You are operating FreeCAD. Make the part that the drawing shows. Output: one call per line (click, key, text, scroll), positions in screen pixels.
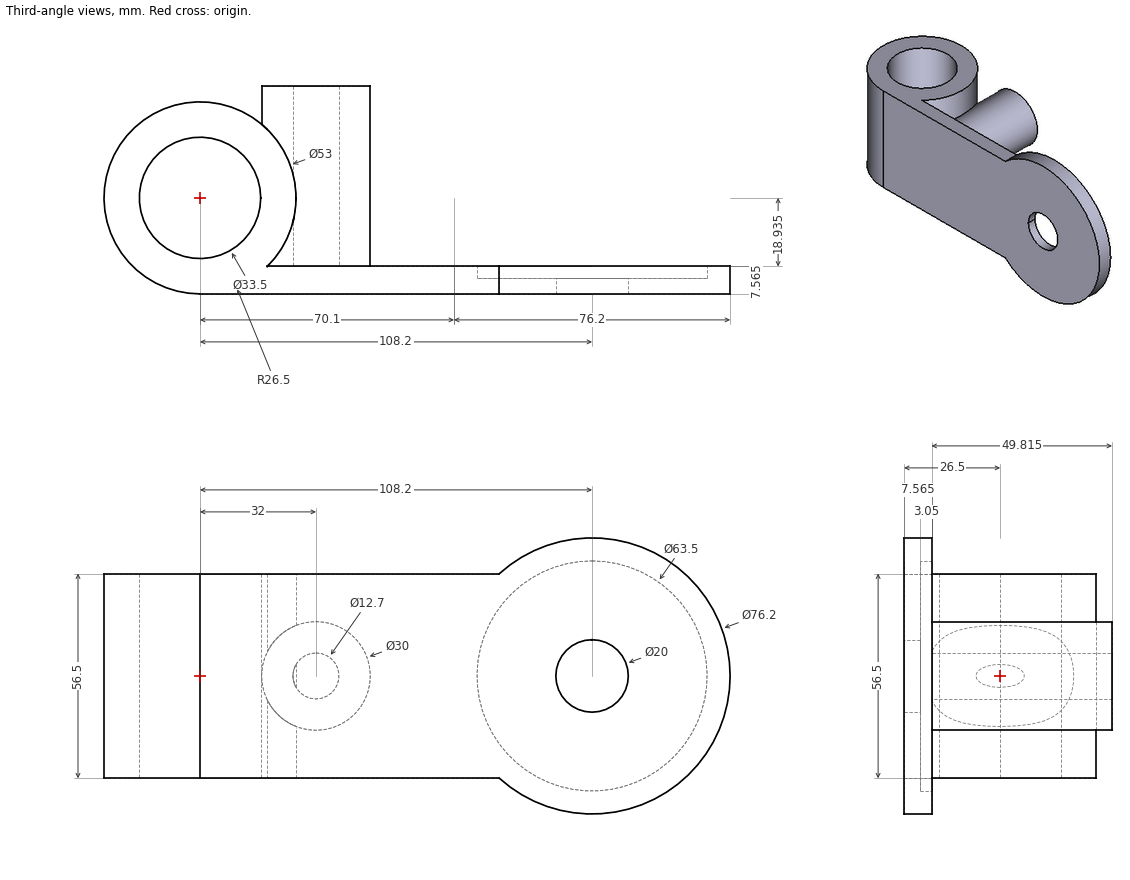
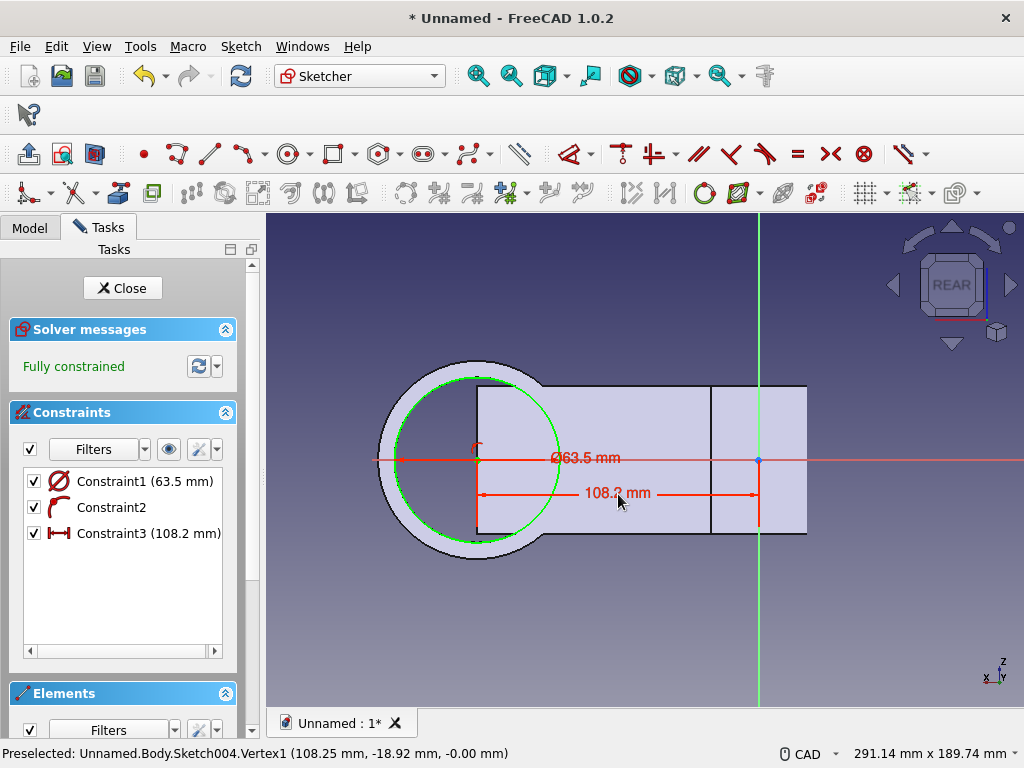
click(123, 288)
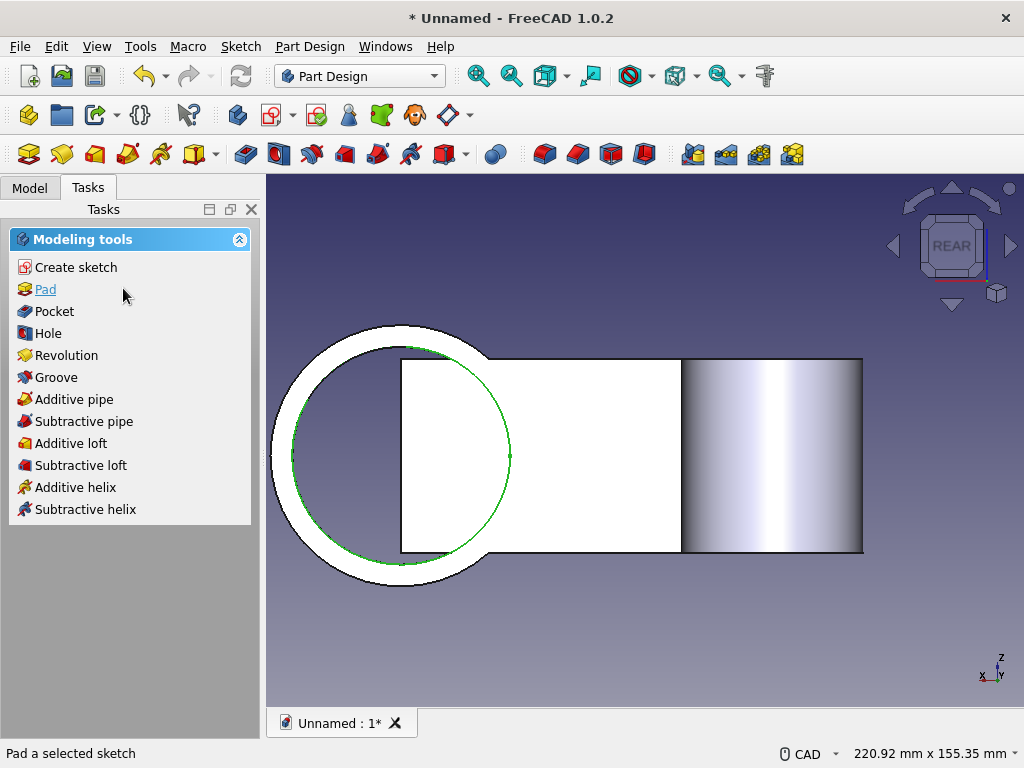
click(29, 154)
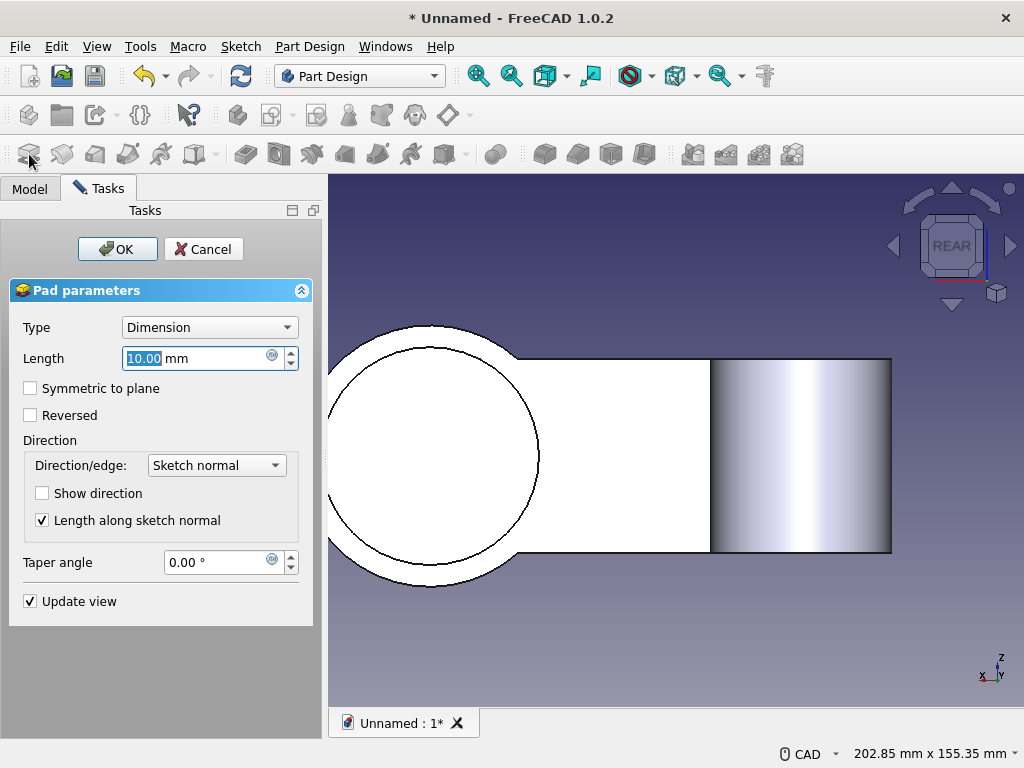
text(7.565)
key(Tab)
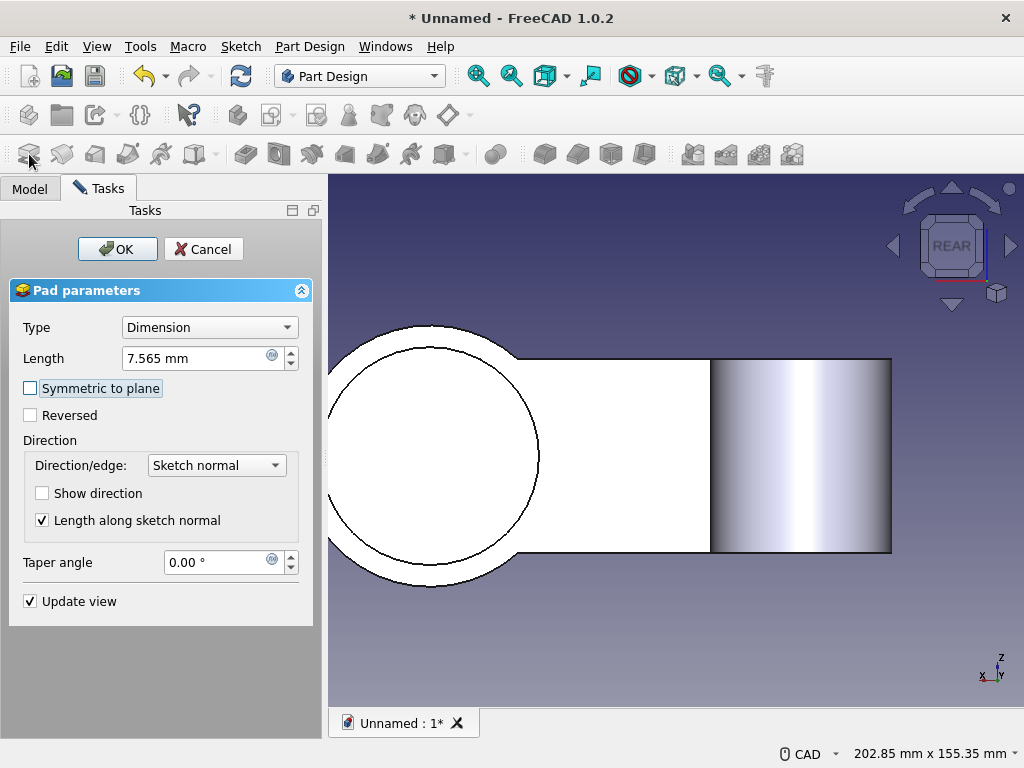
click(31, 415)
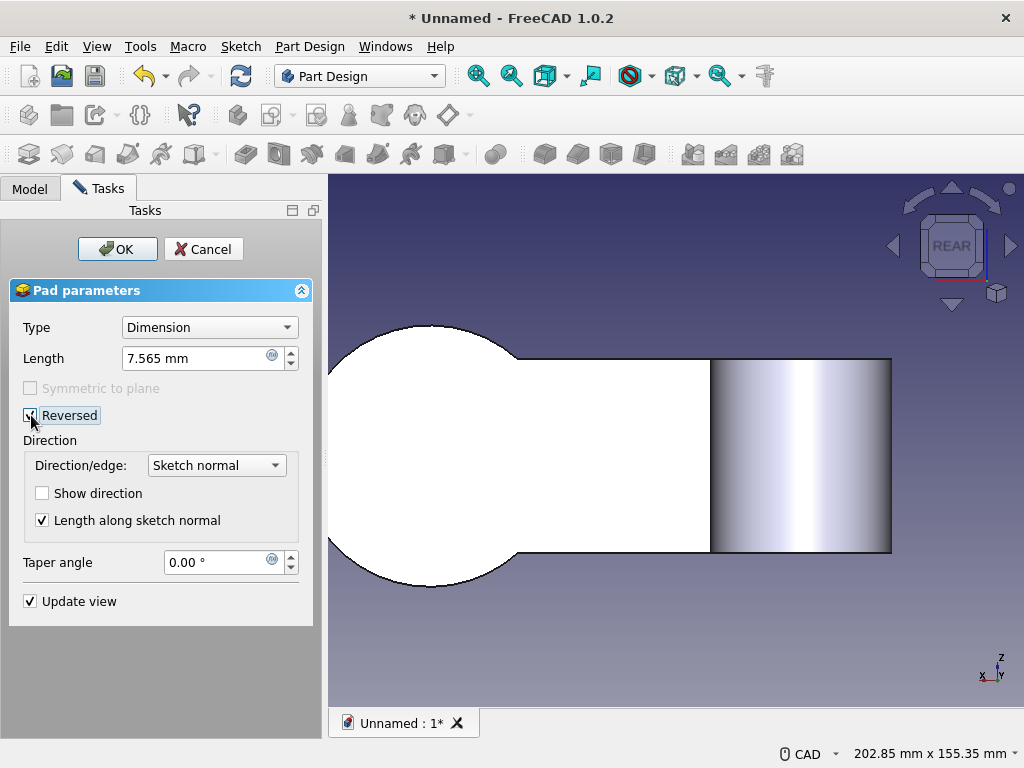
click(118, 249)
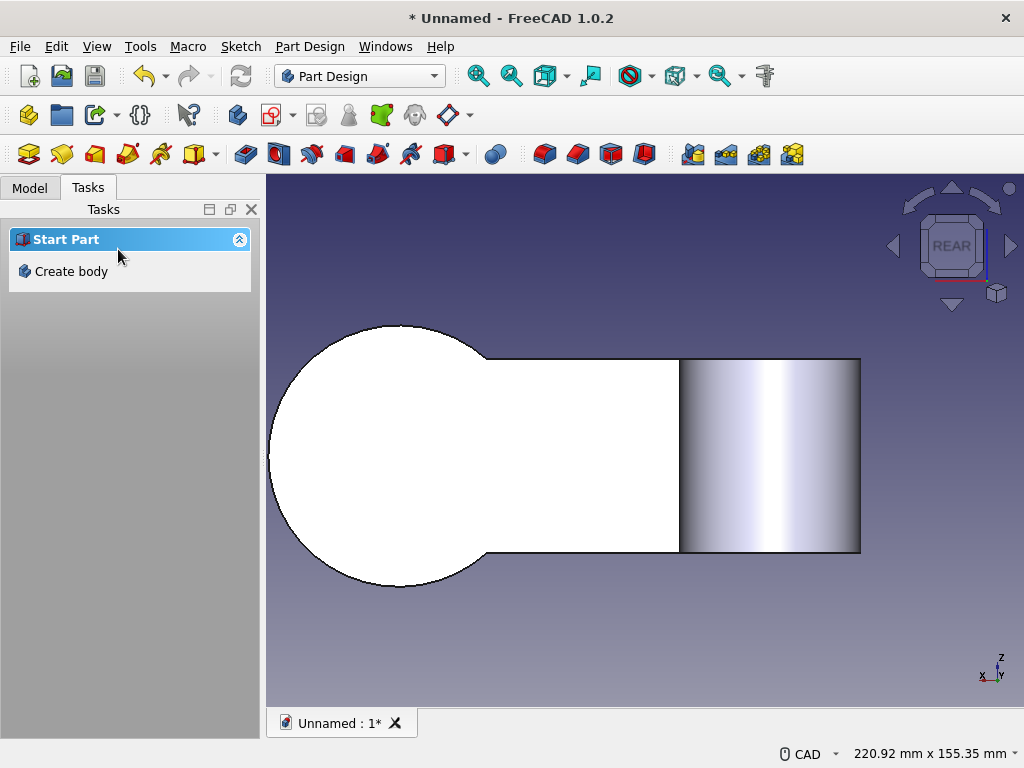
click(425, 455)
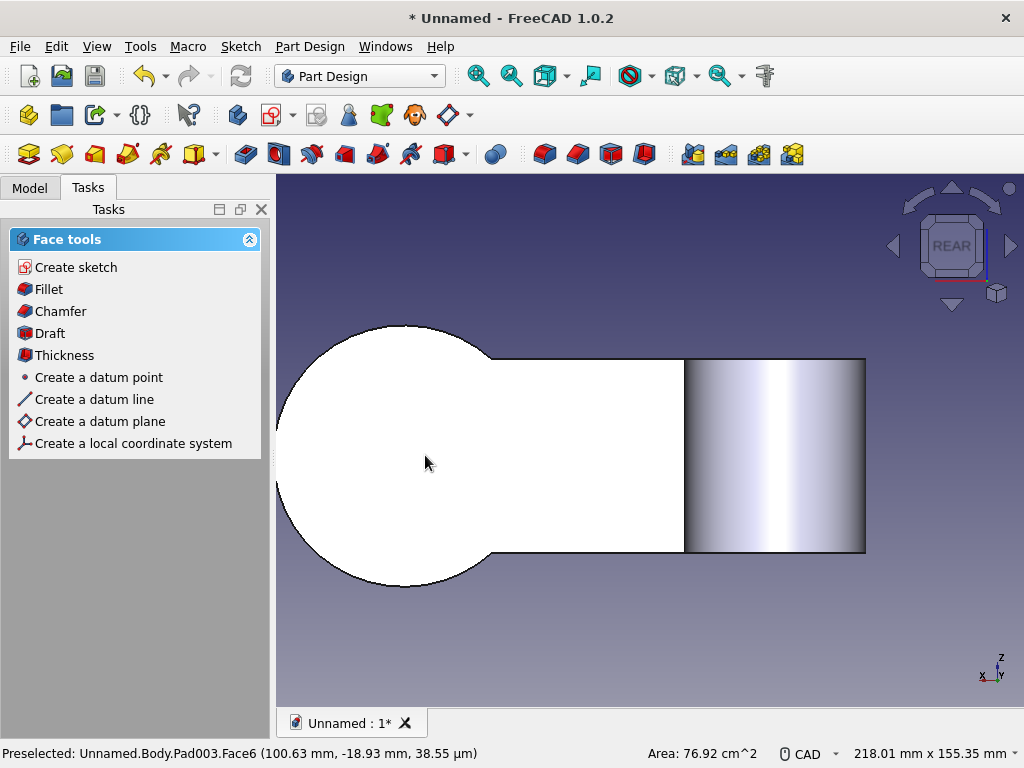
click(270, 116)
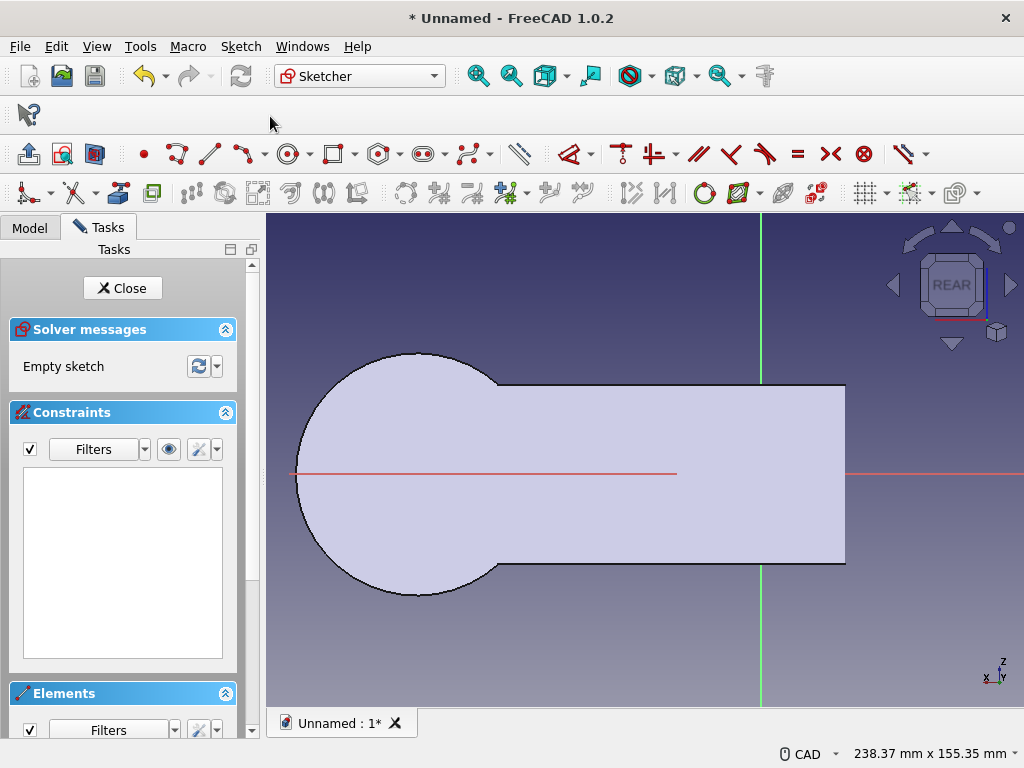
scroll(748, 395, down, 1)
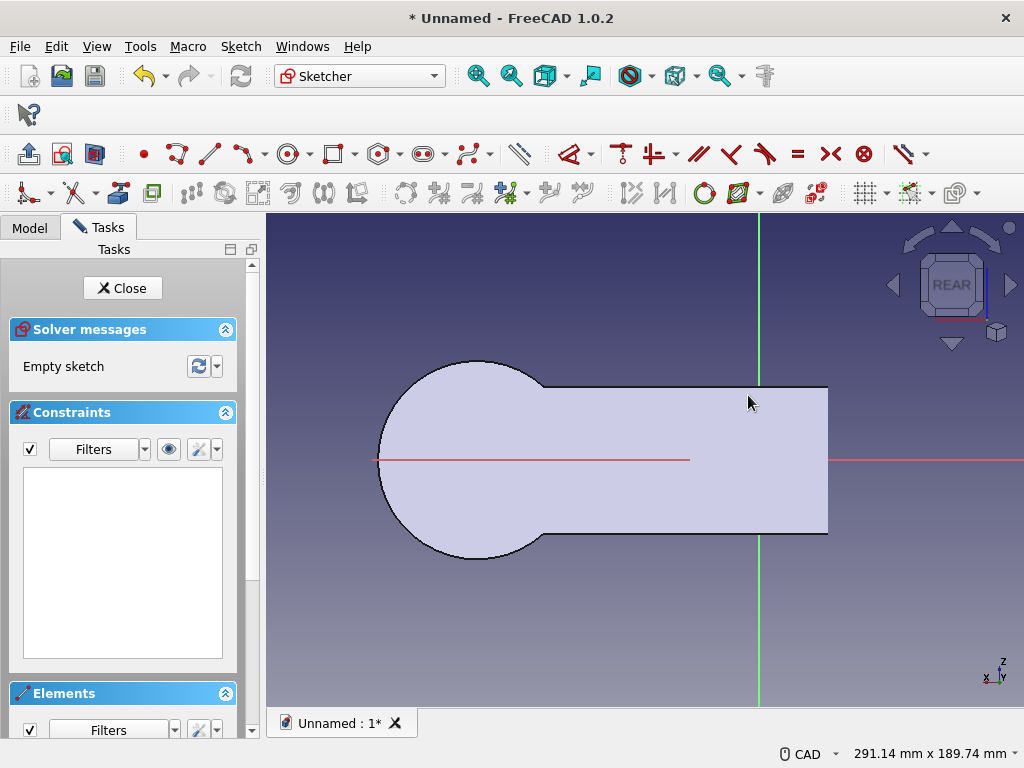
key(g)
key(c)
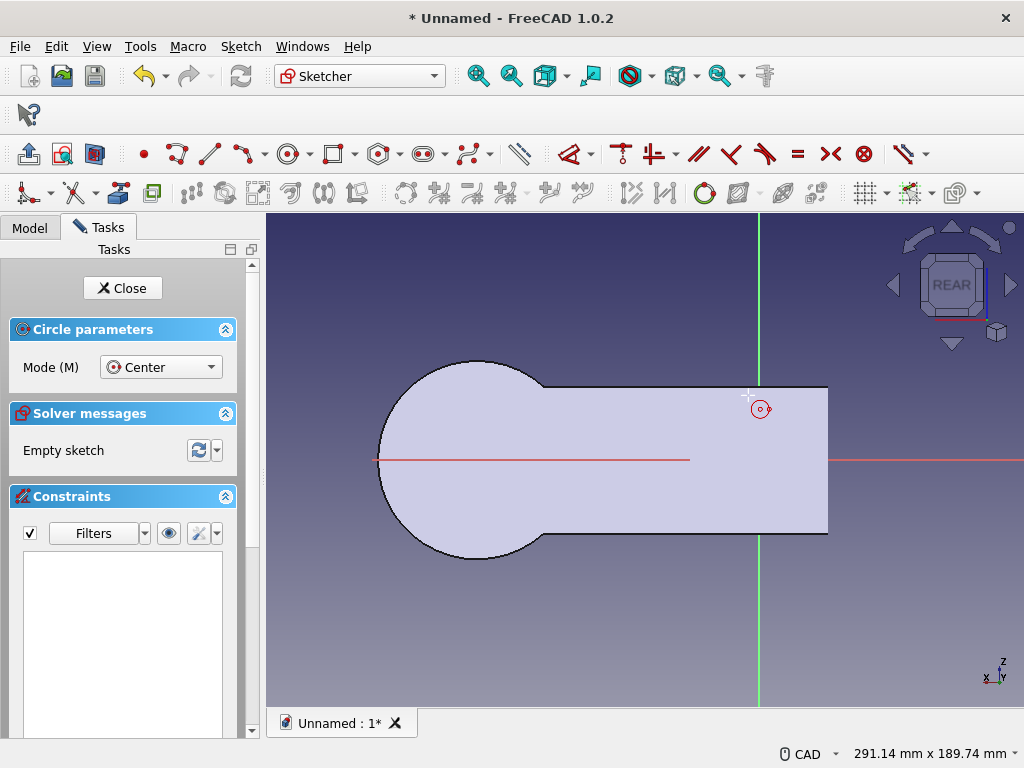
click(477, 460)
move(536, 402)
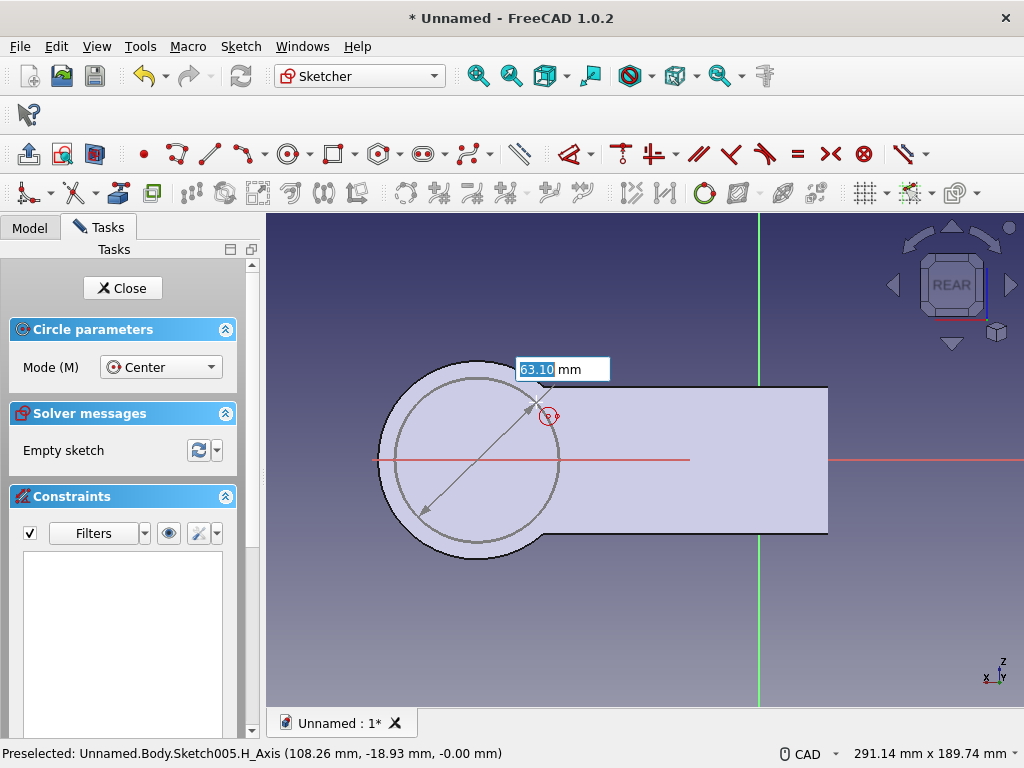
text(63.5)
key(Return)
key(Escape)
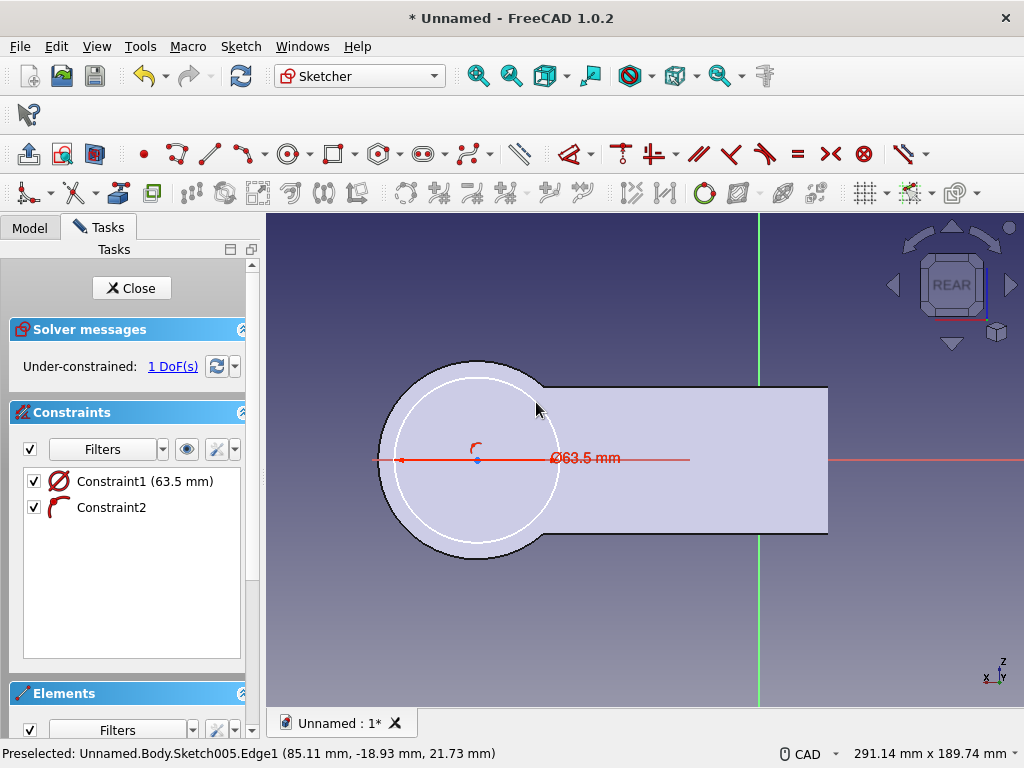
key(d)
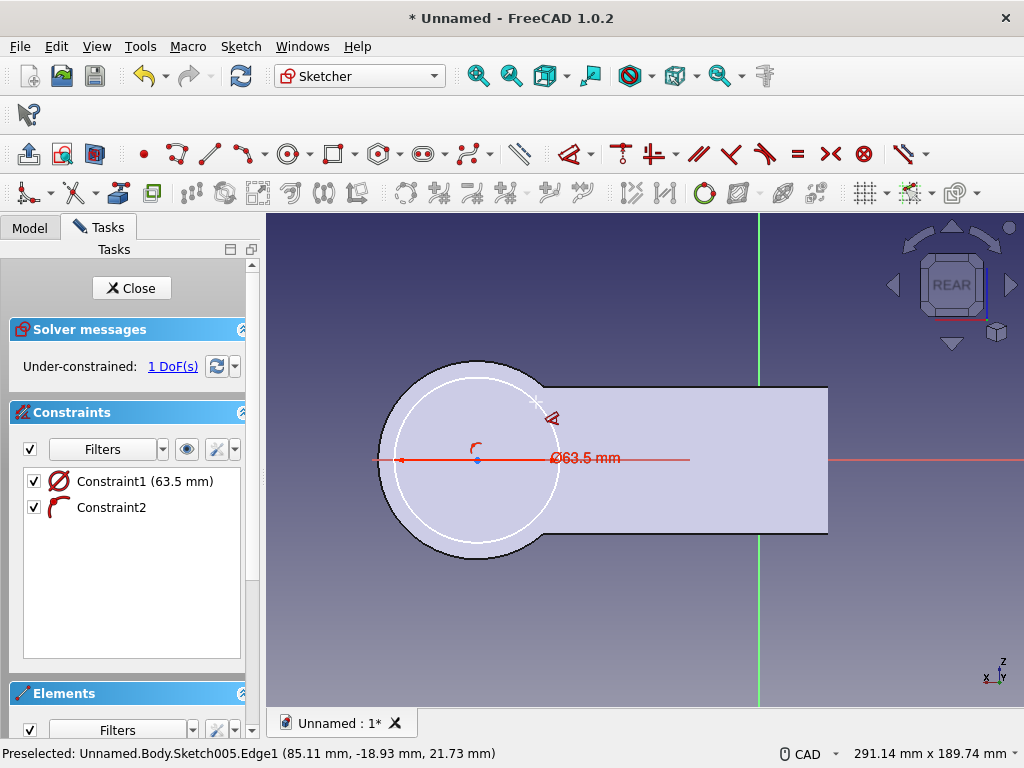
click(477, 460)
click(618, 494)